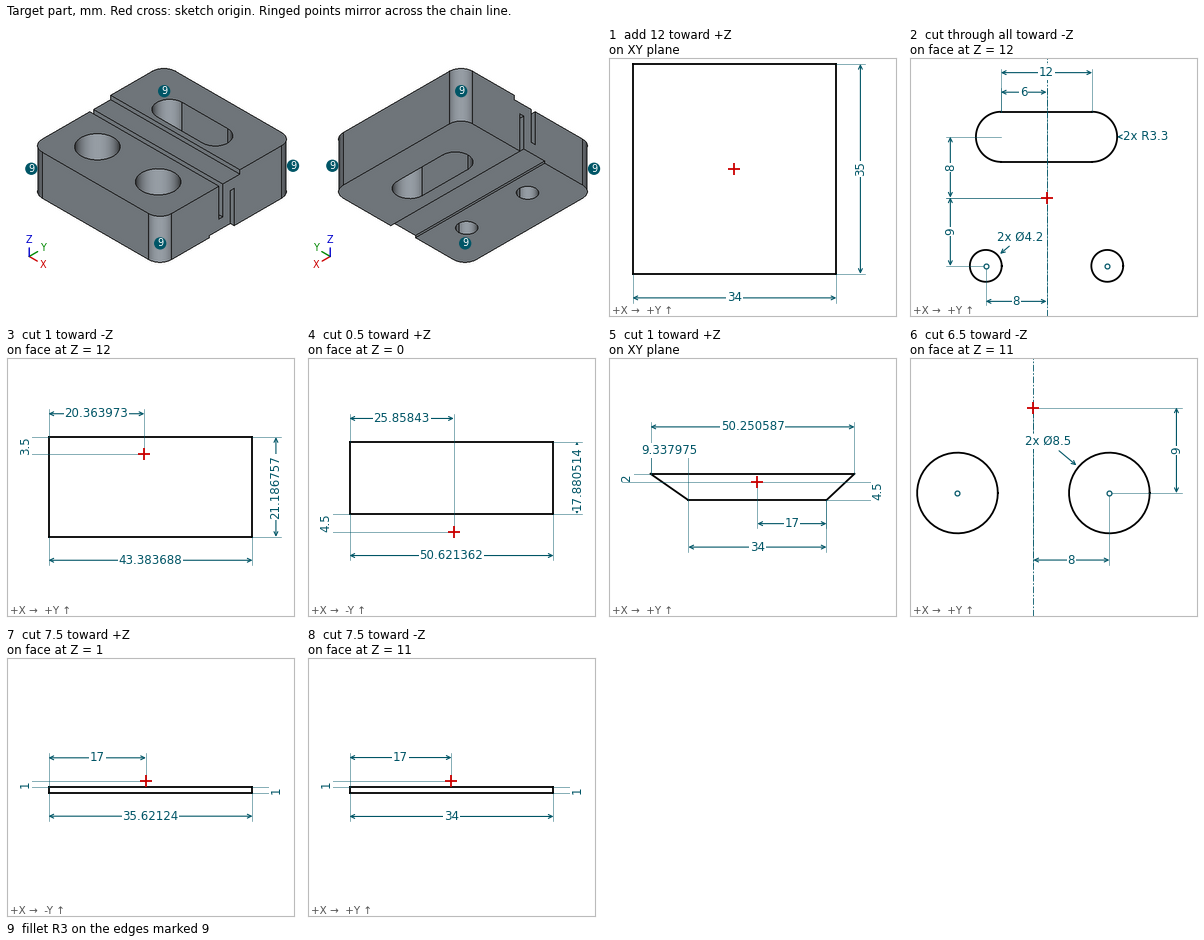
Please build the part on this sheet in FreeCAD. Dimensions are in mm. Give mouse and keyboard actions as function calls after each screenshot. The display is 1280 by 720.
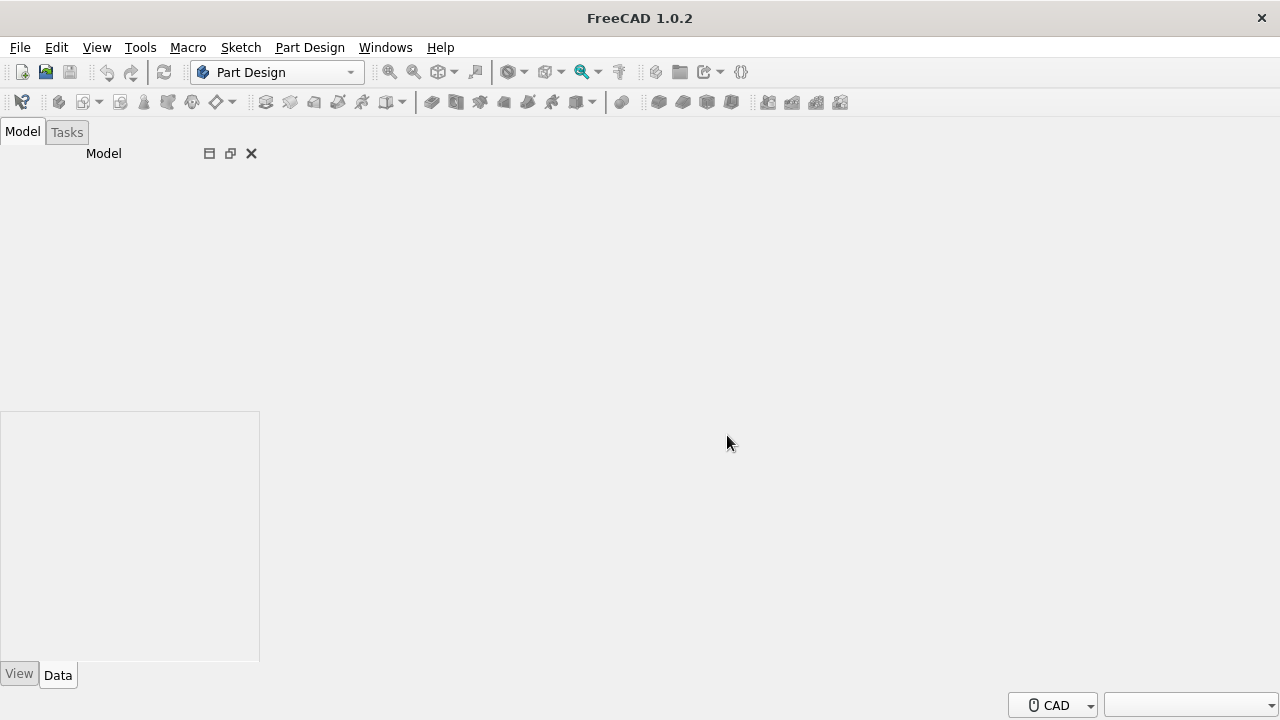
key(ctrl+n)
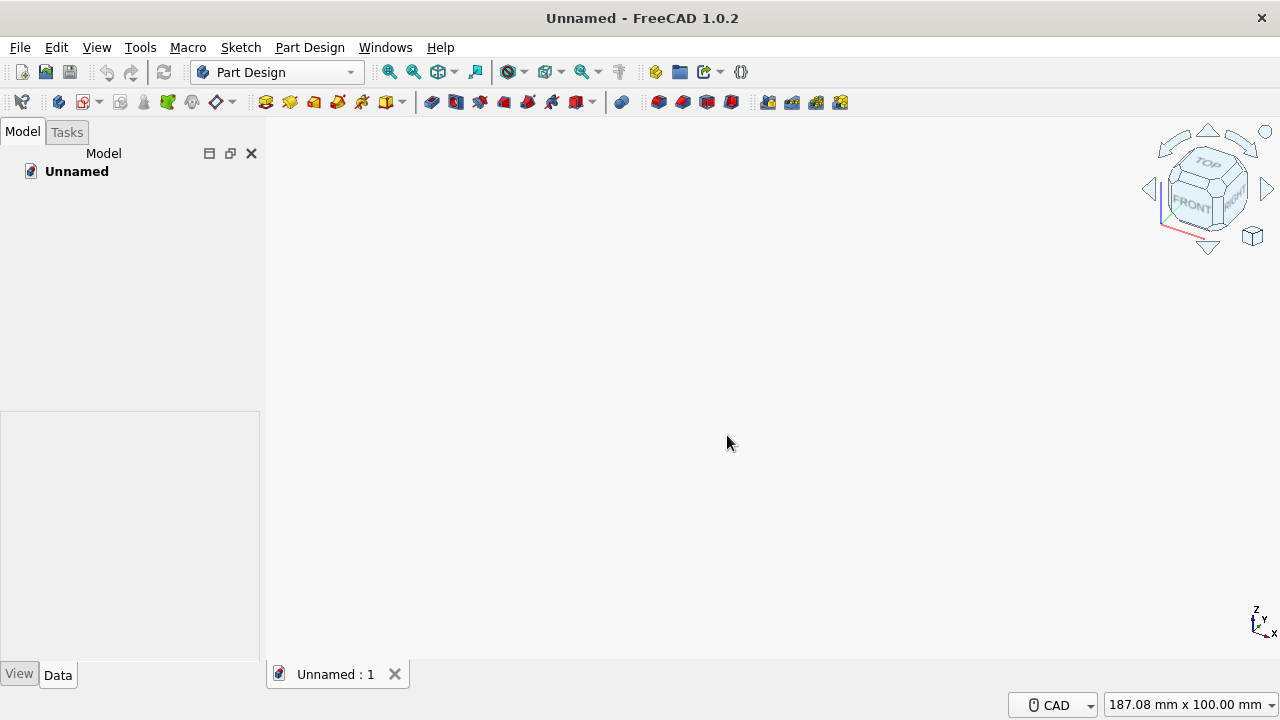
click(84, 102)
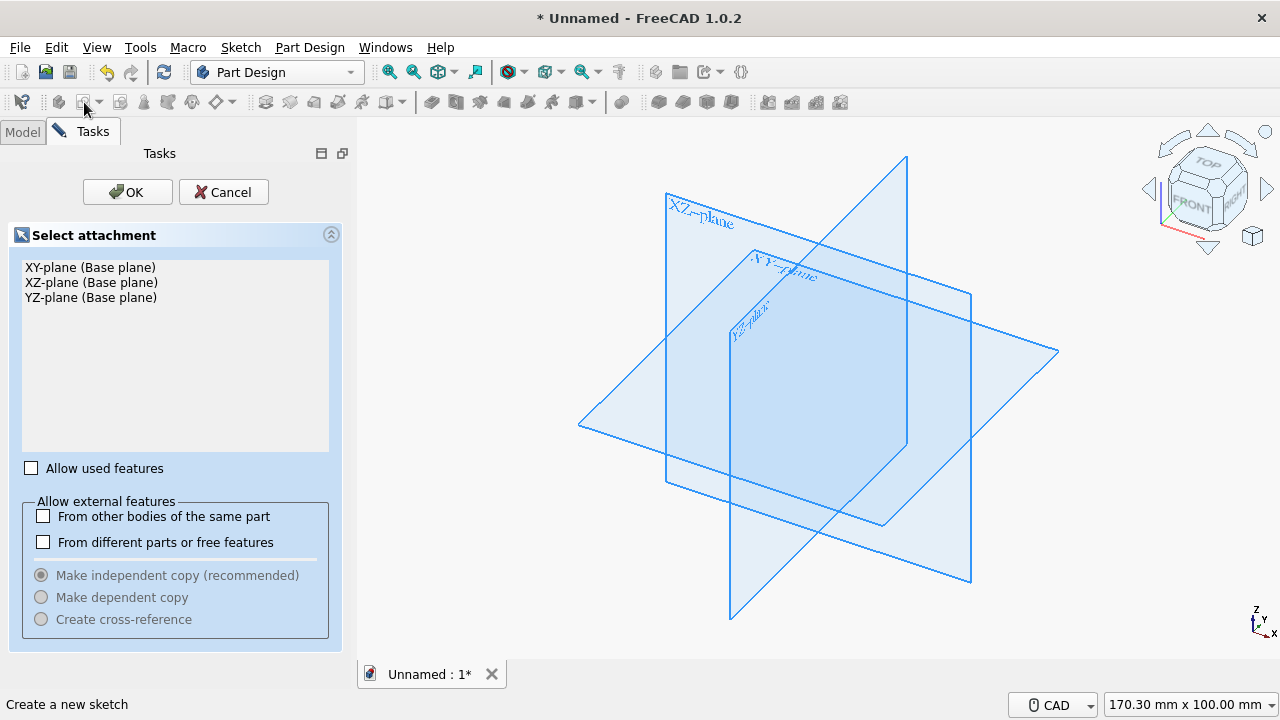
click(82, 268)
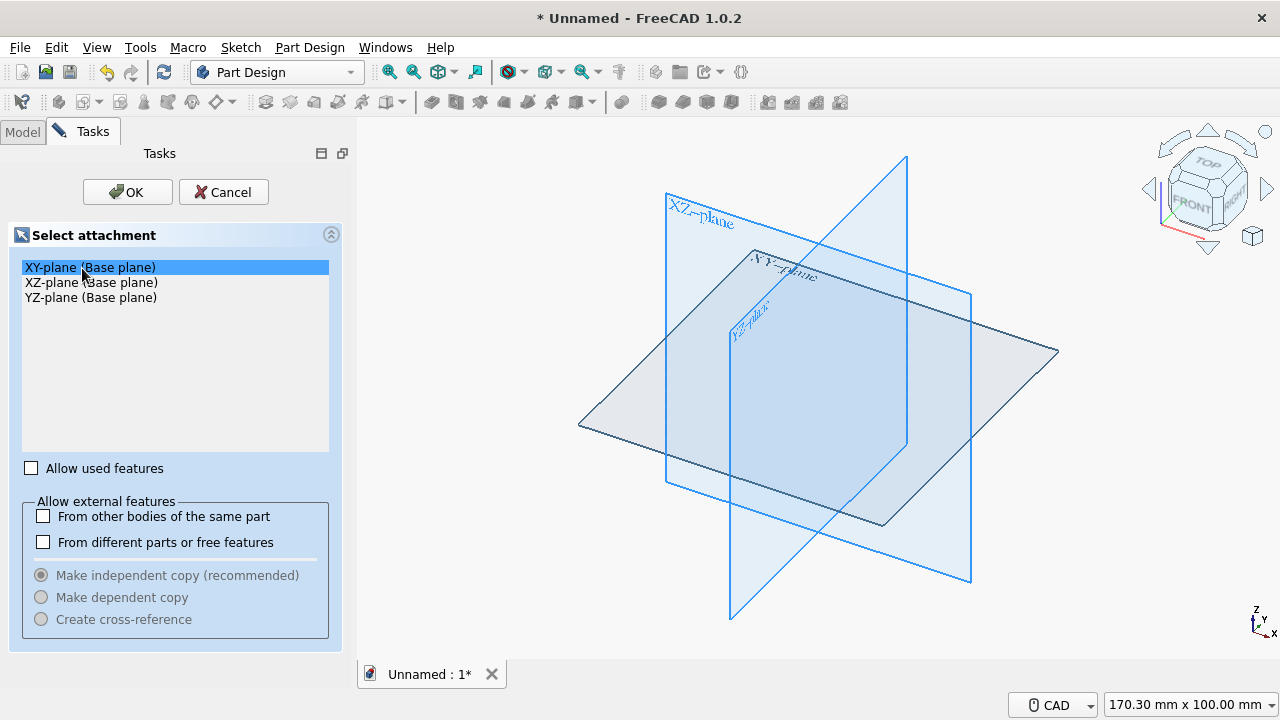
click(128, 192)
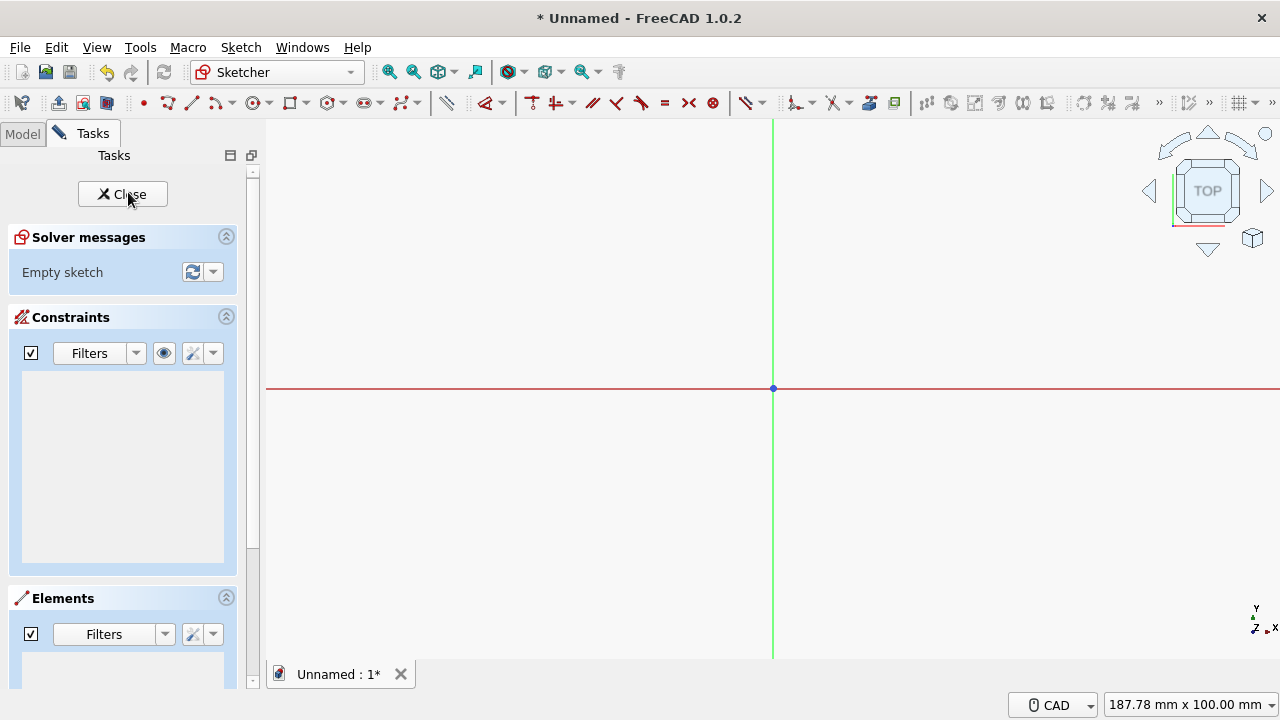
scroll(856, 389, up, 3)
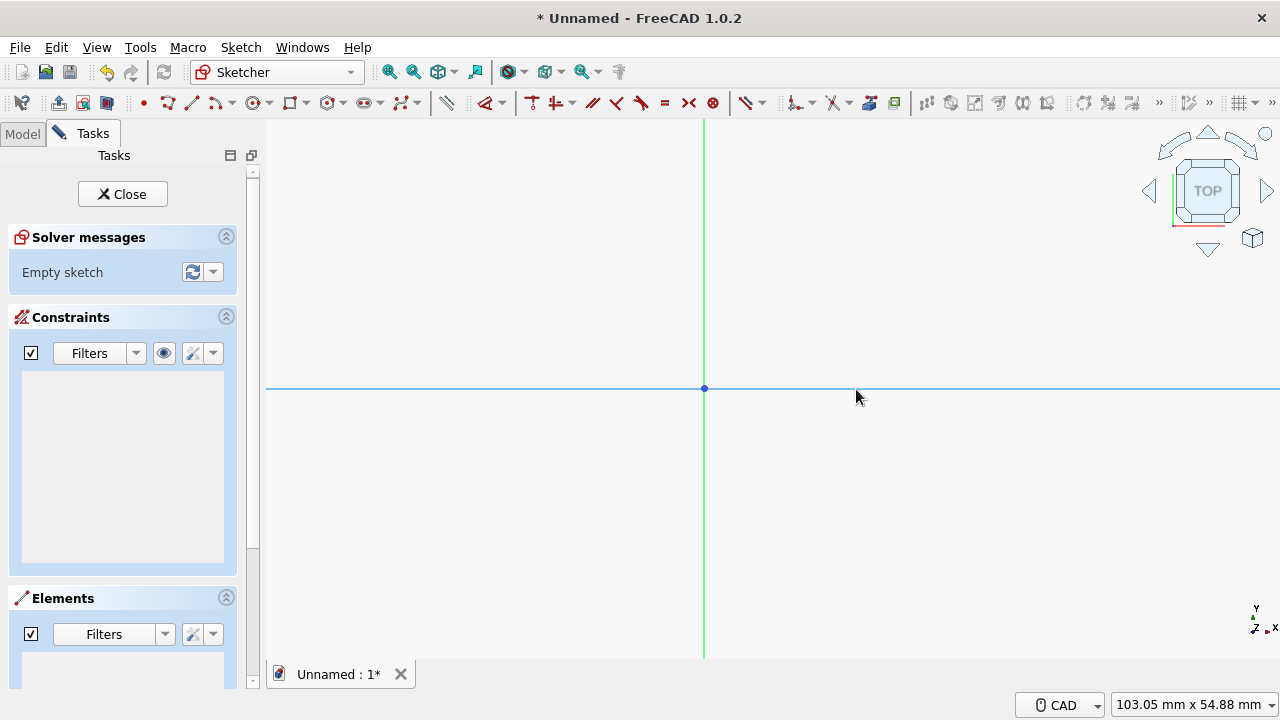
key(g)
key(v)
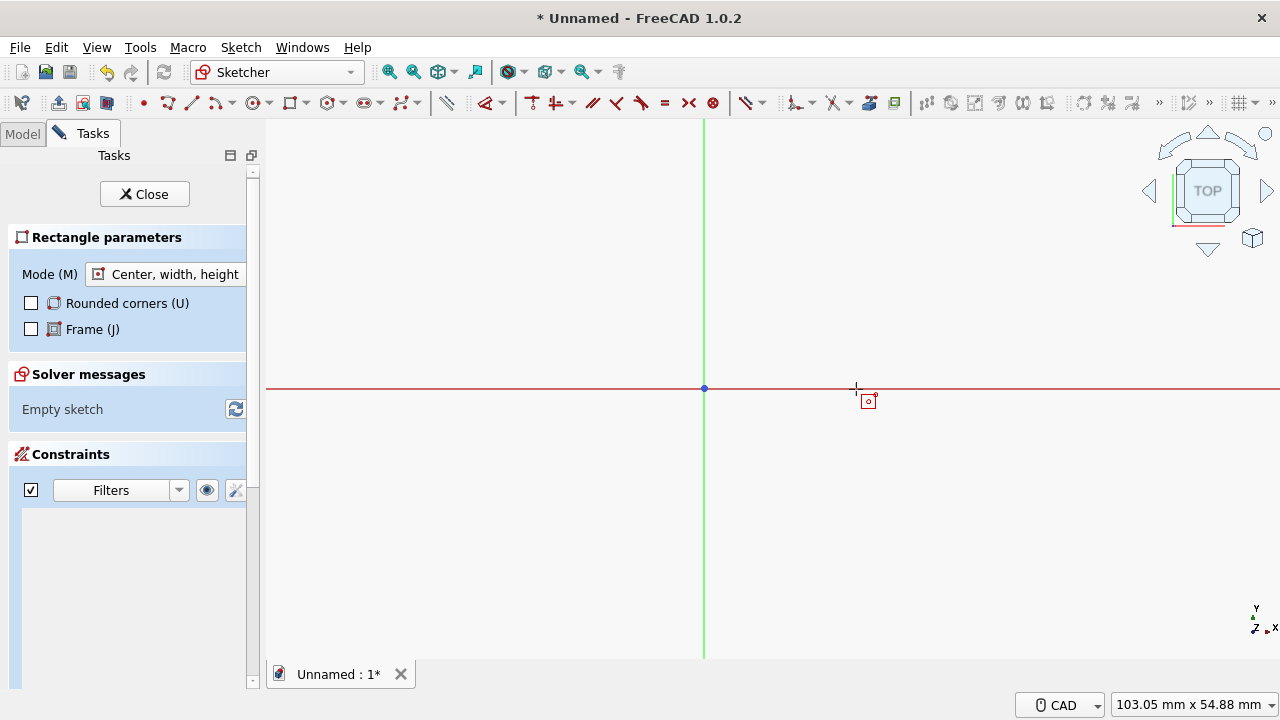
click(704, 389)
move(872, 216)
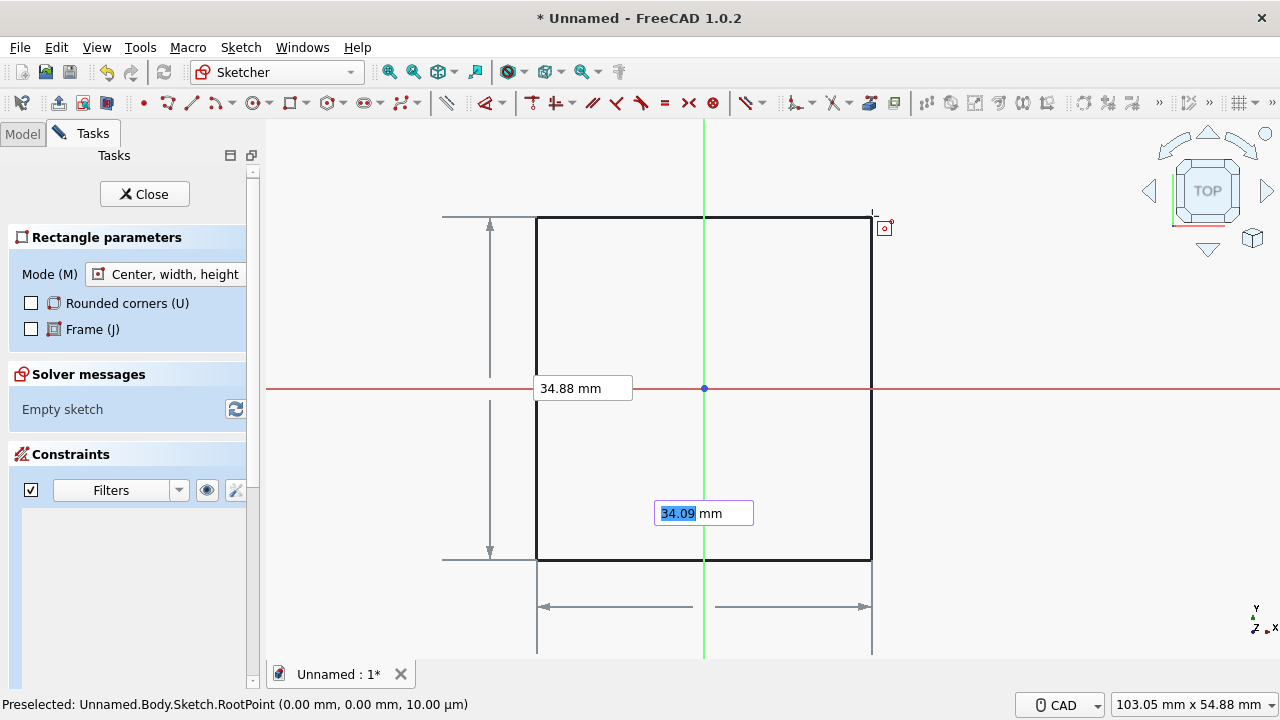
text(34)
key(Tab)
text(35)
key(Return)
key(Escape)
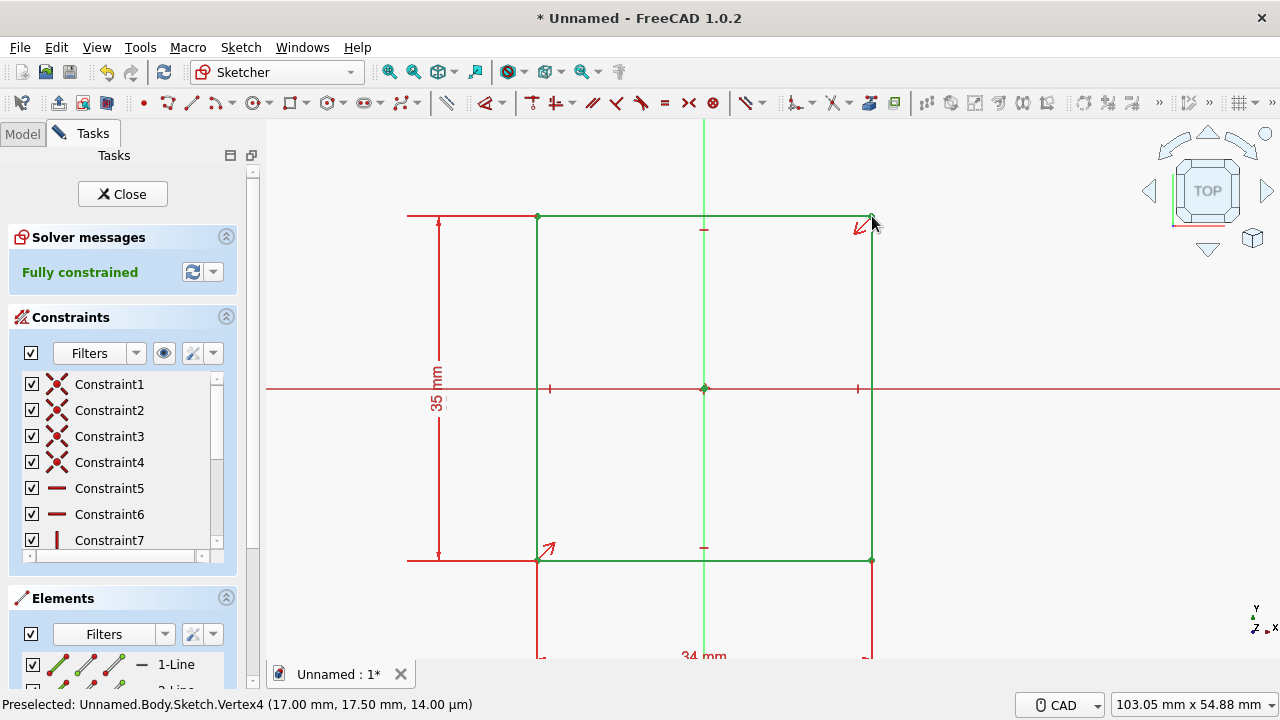
click(123, 194)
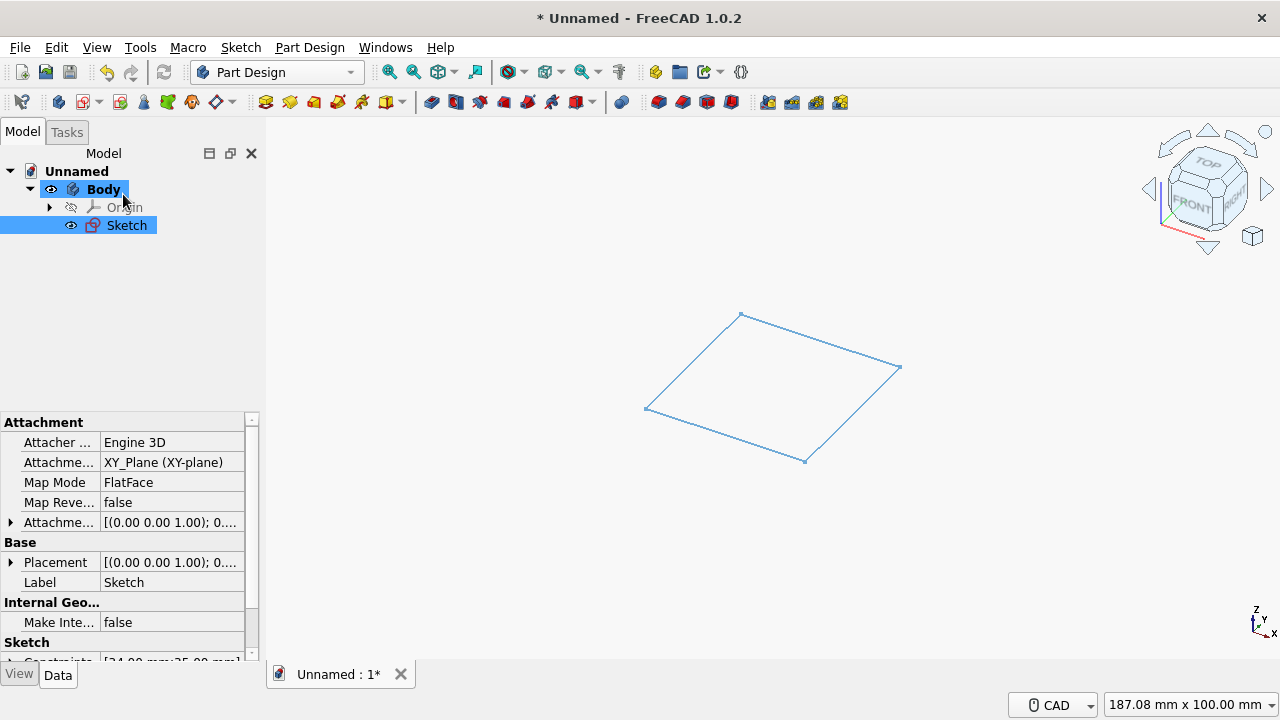
click(266, 102)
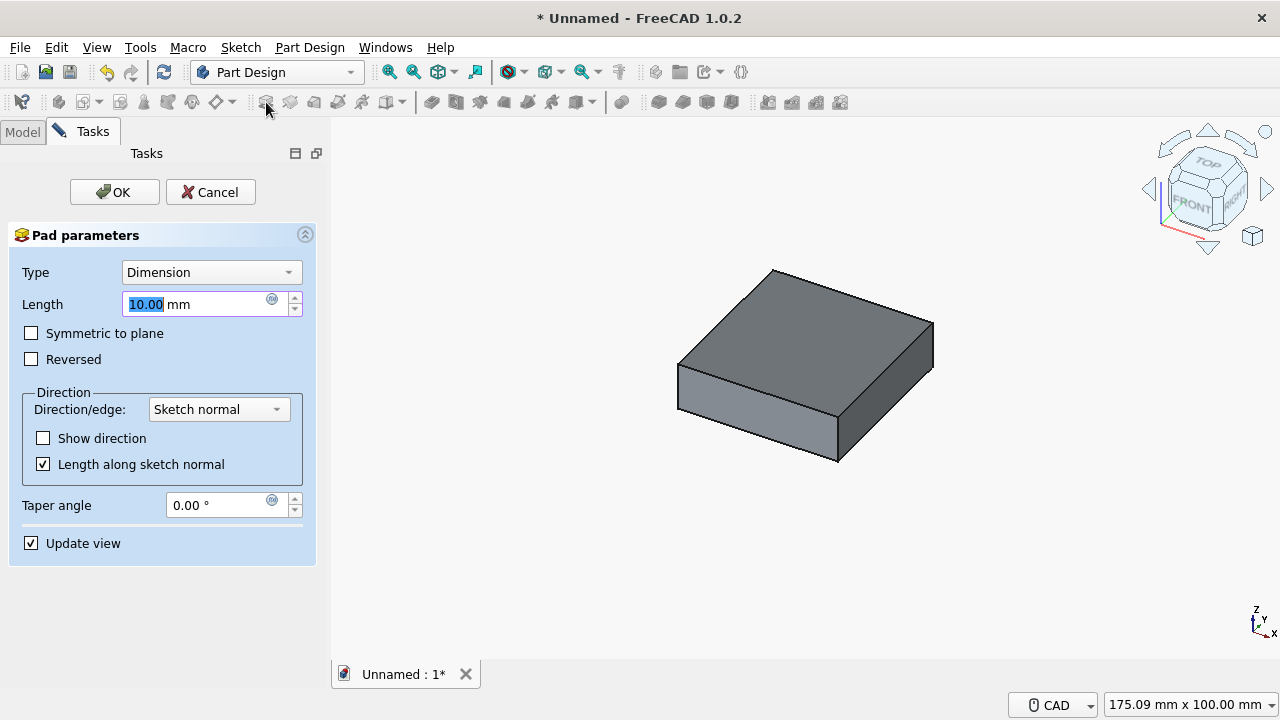
text(12)
key(Tab)